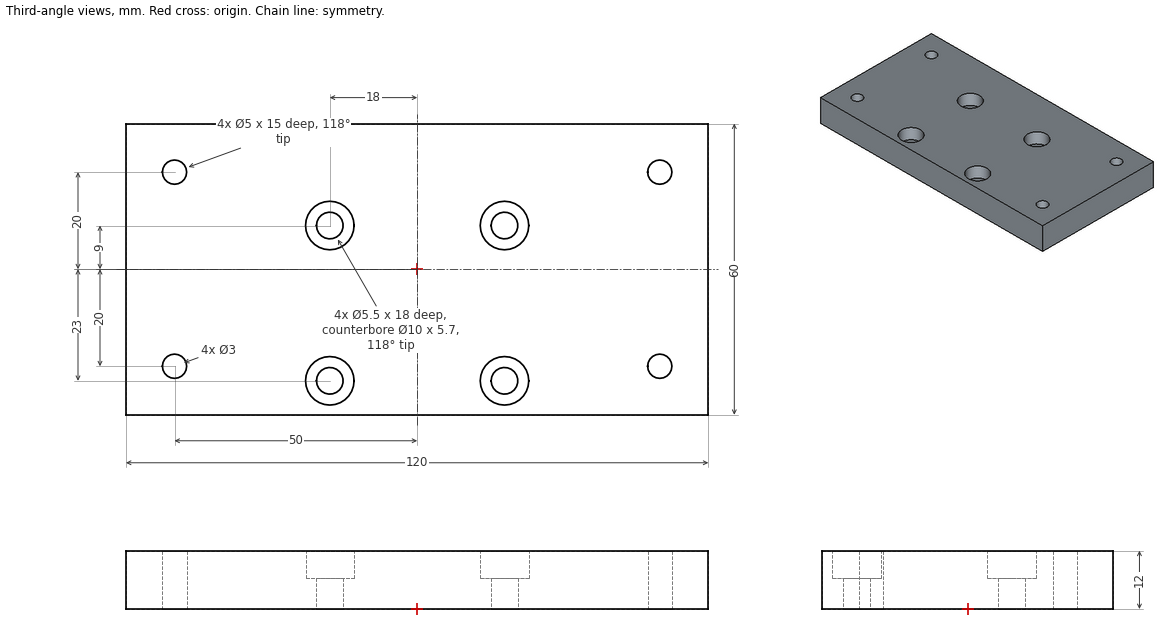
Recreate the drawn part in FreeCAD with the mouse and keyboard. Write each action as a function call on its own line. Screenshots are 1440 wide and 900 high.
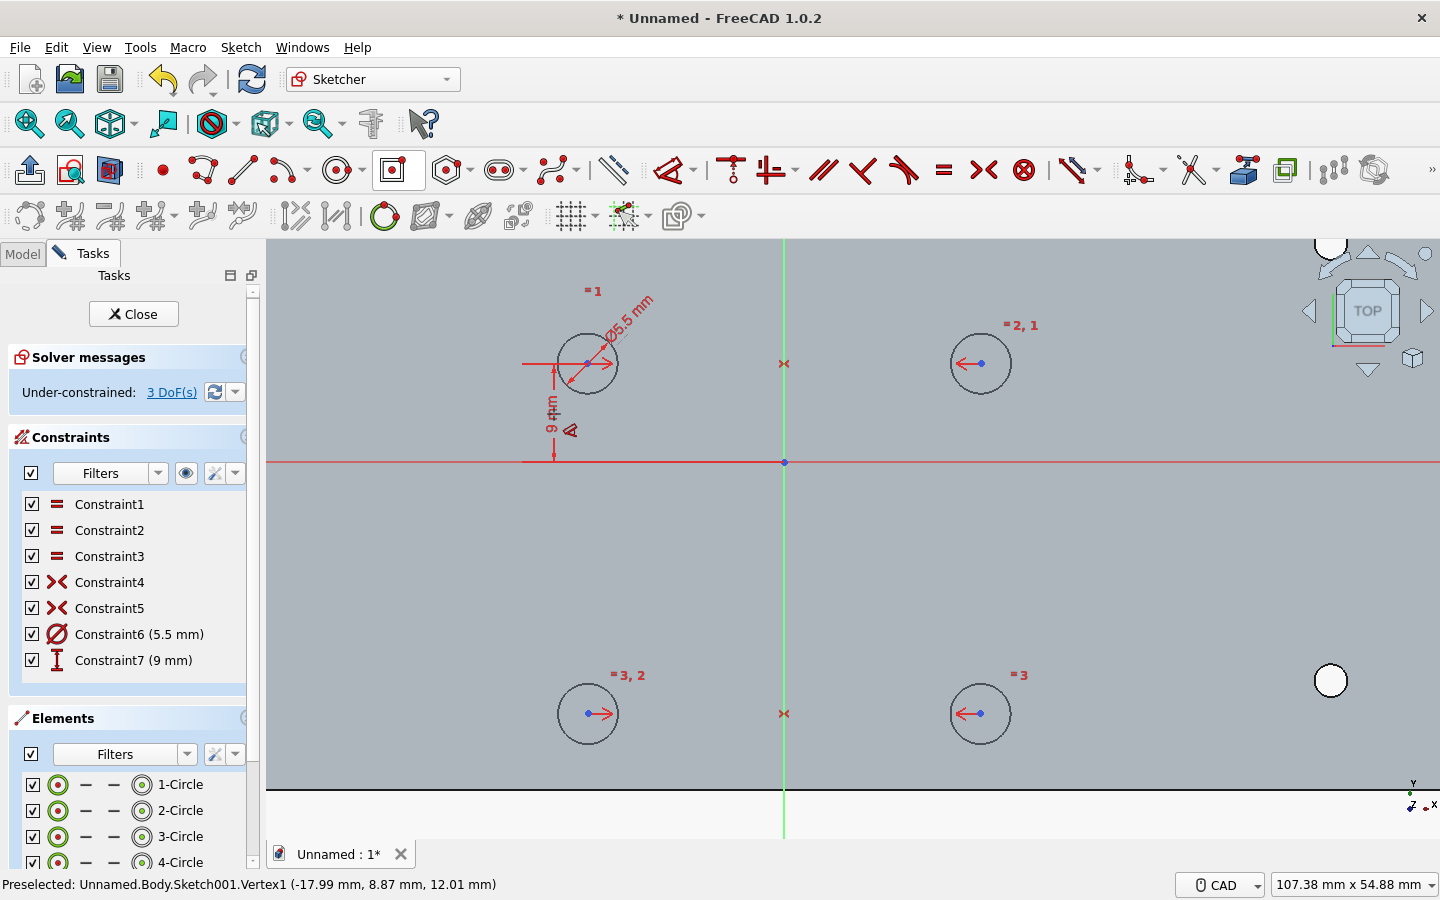
click(588, 364)
click(731, 330)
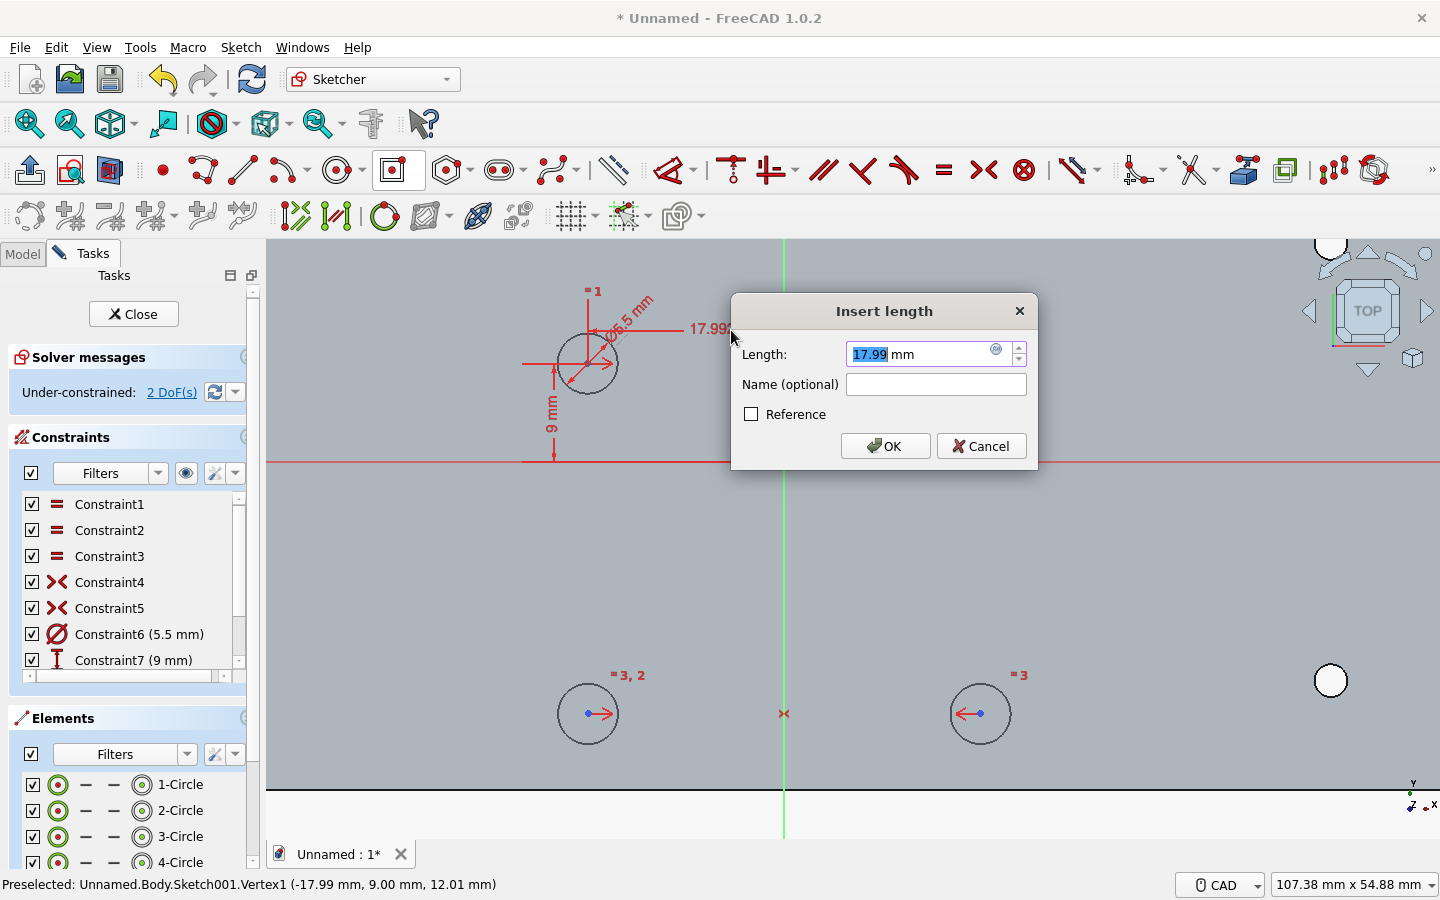
text(18)
key(Return)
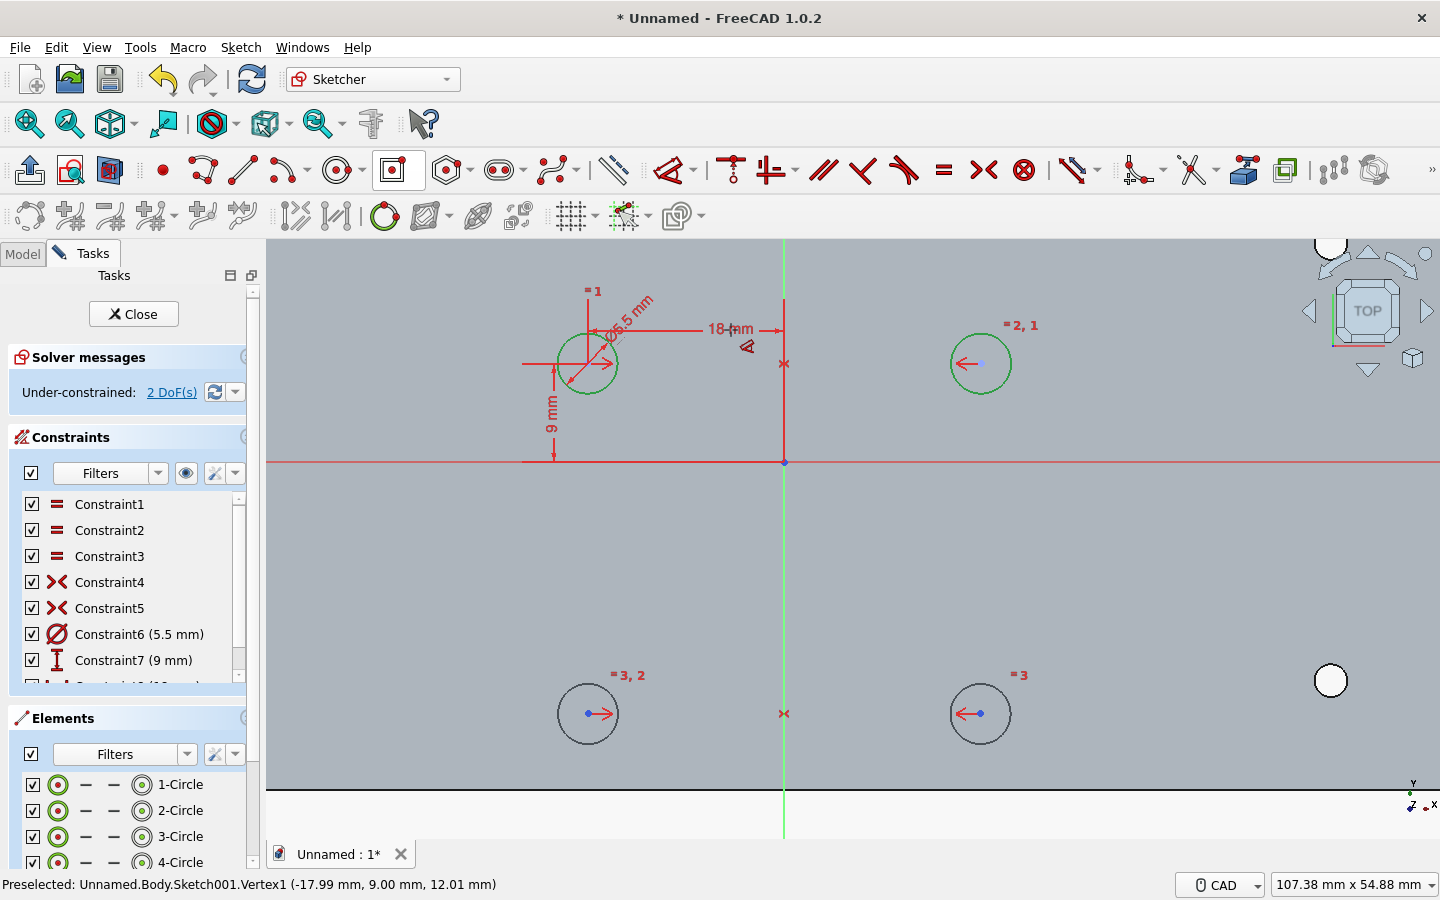
click(588, 714)
click(686, 748)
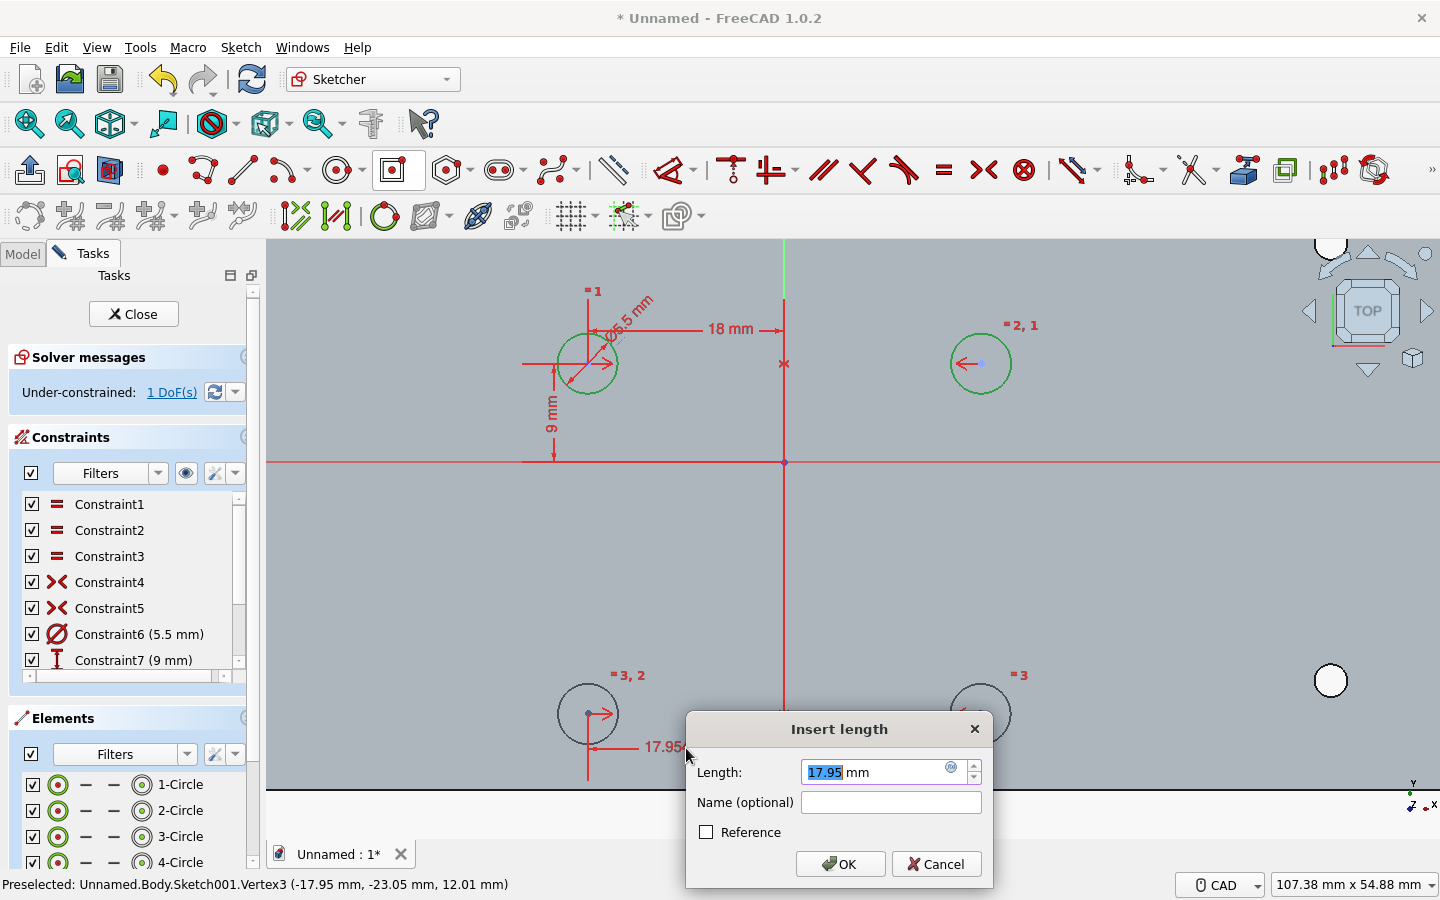
text(18)
key(Return)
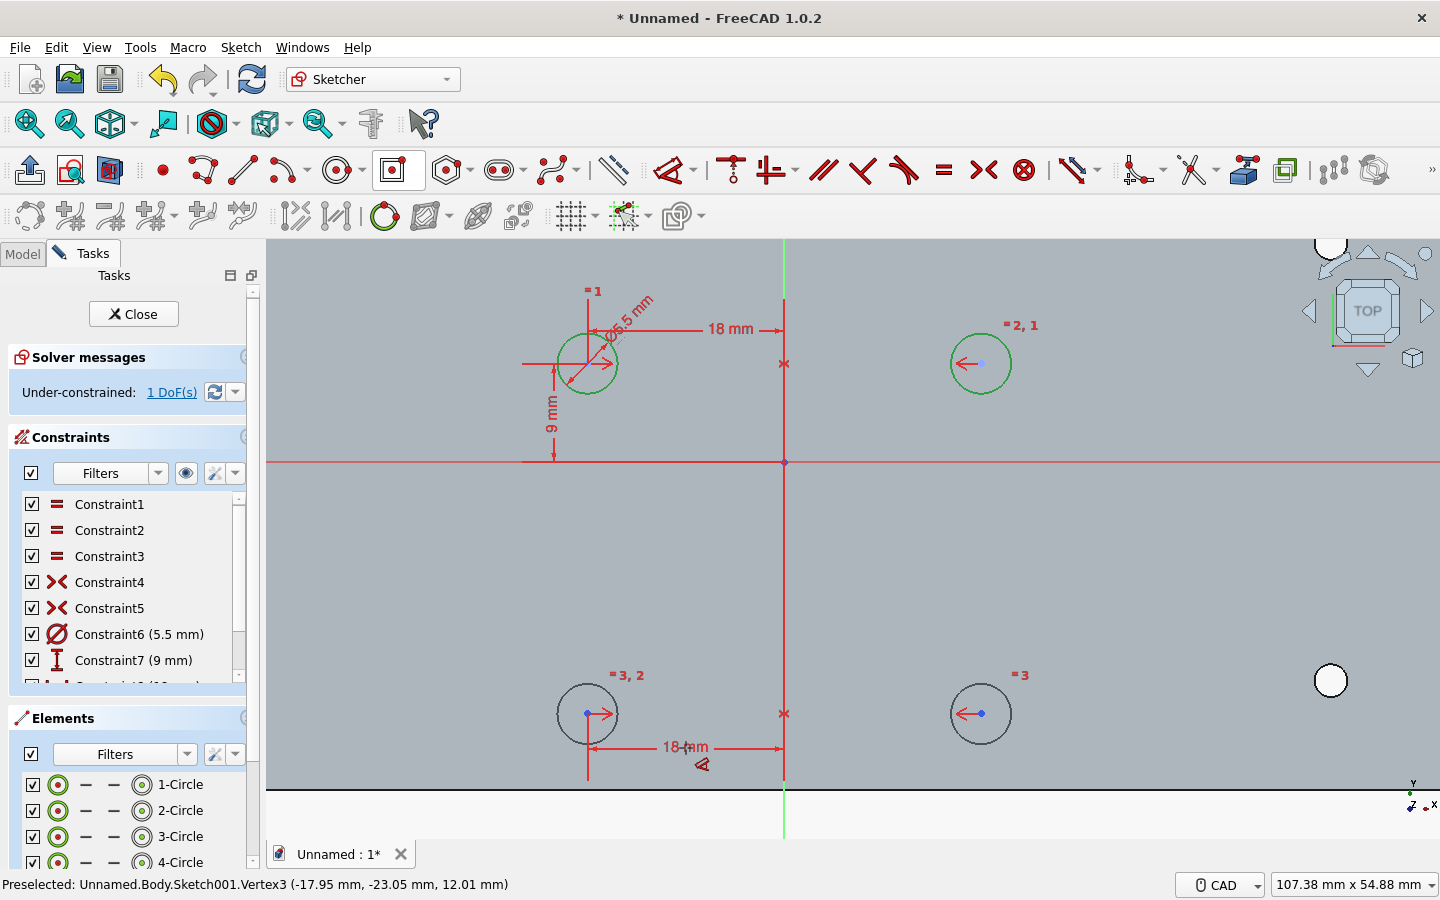
click(588, 714)
click(554, 588)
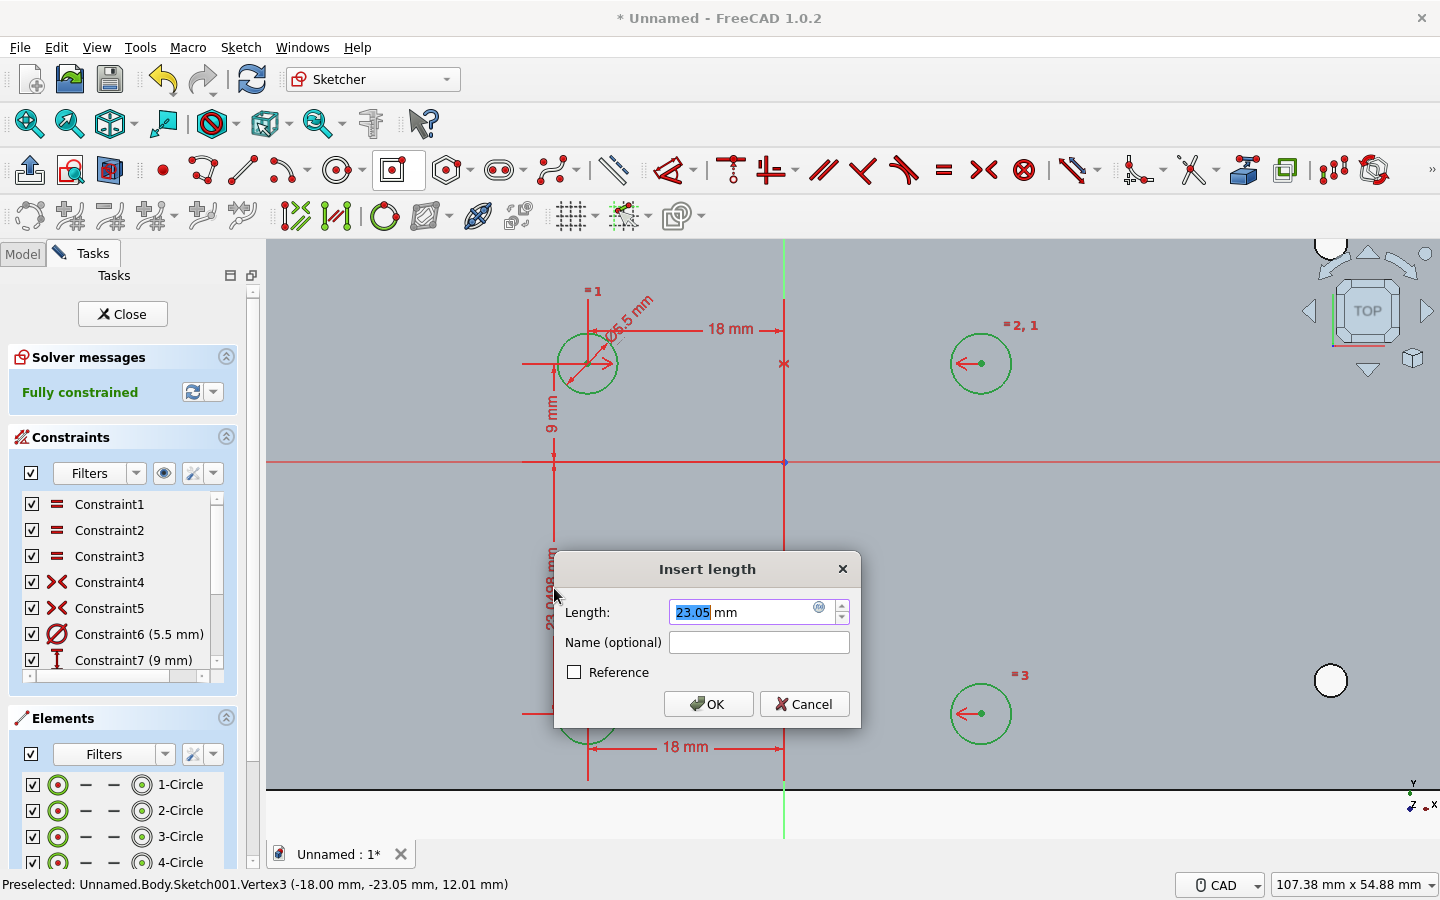
text(23)
key(Return)
key(Escape)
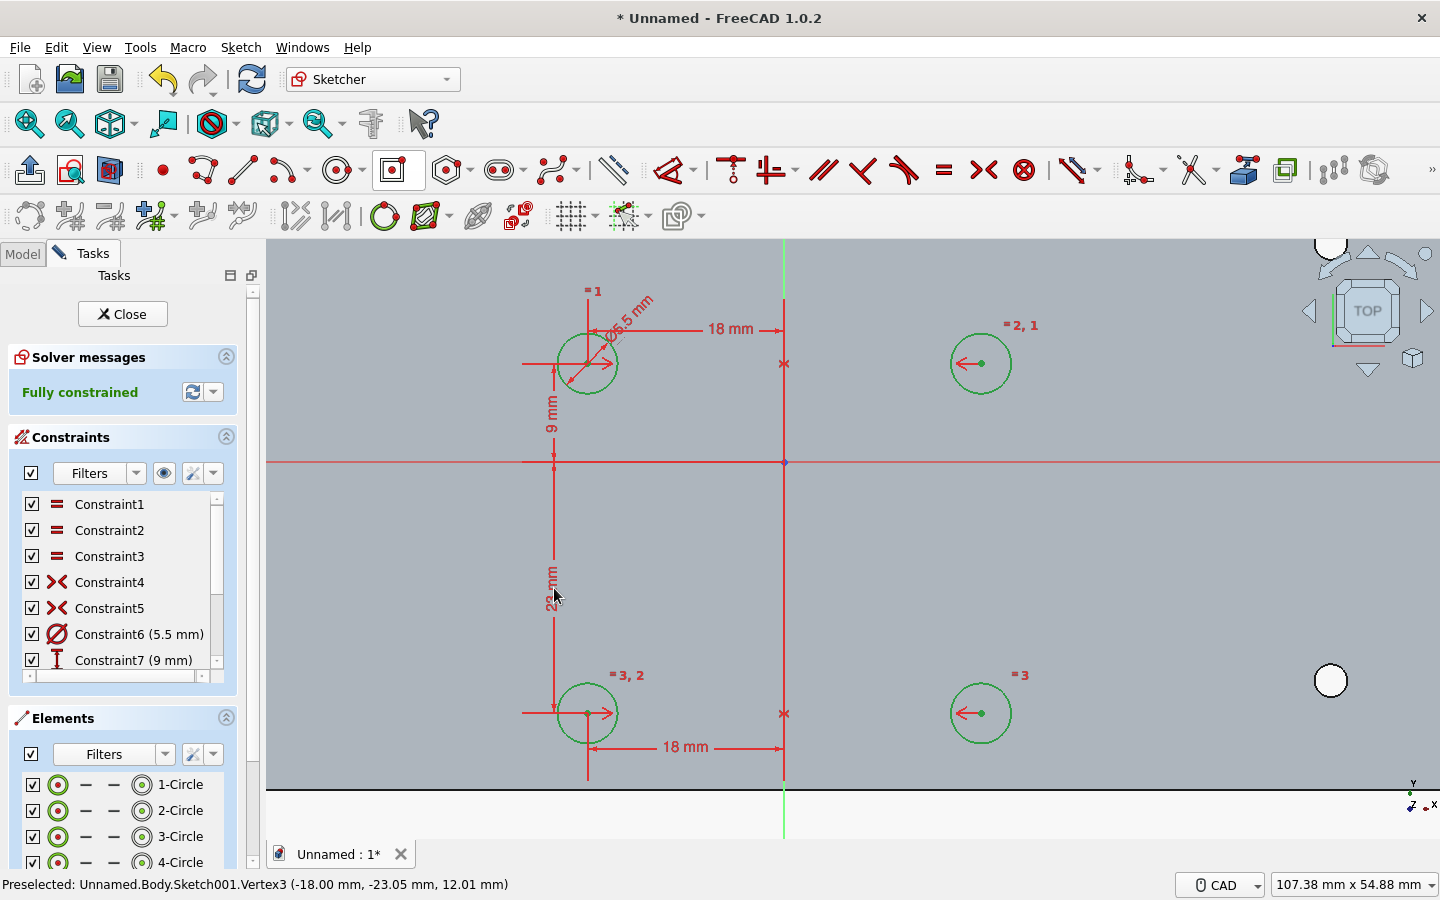
click(123, 314)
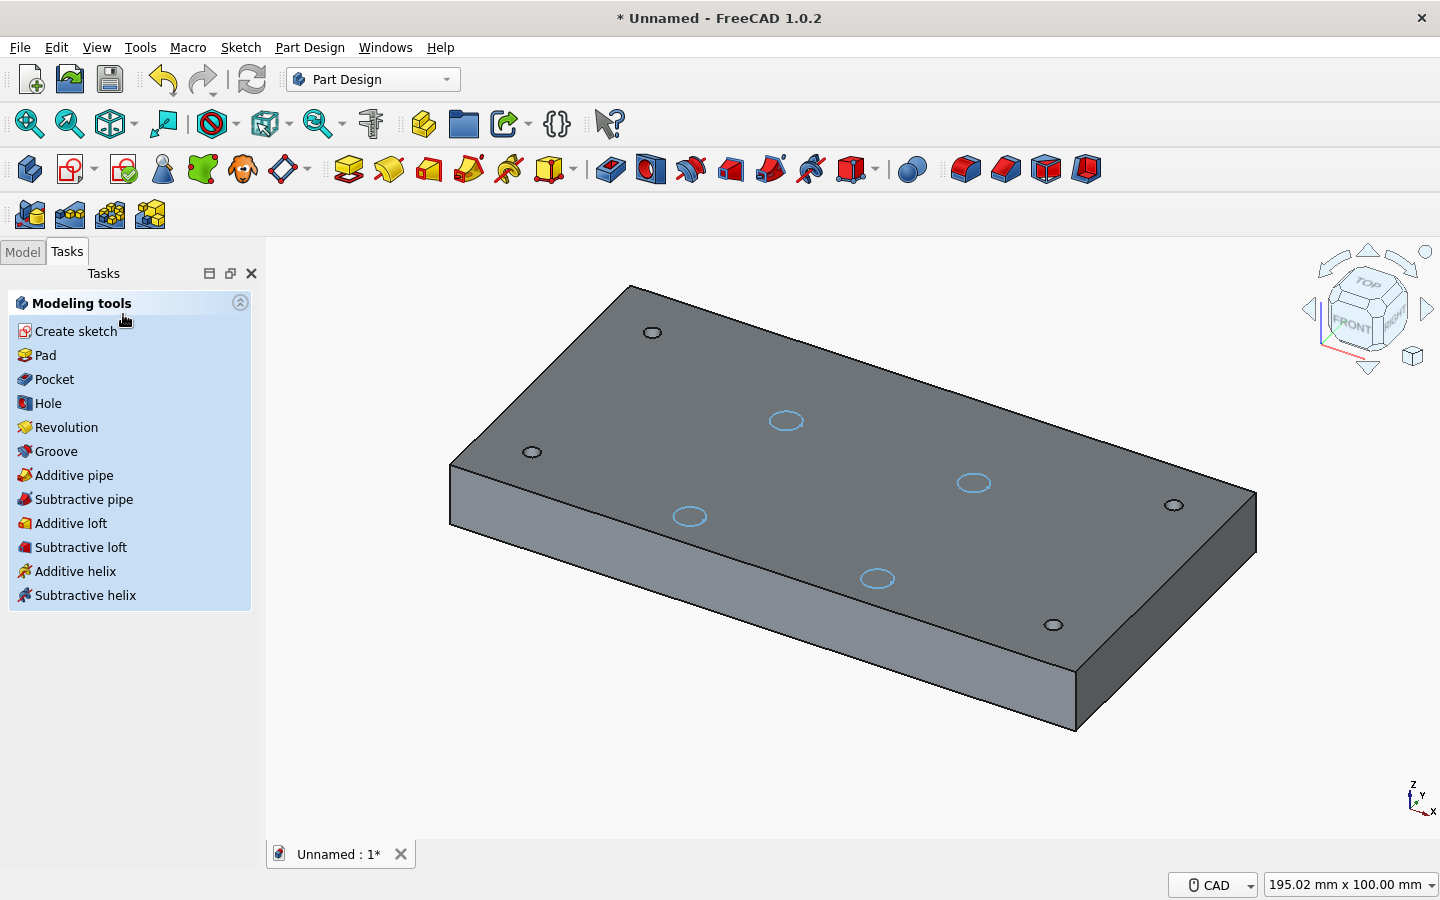
click(652, 170)